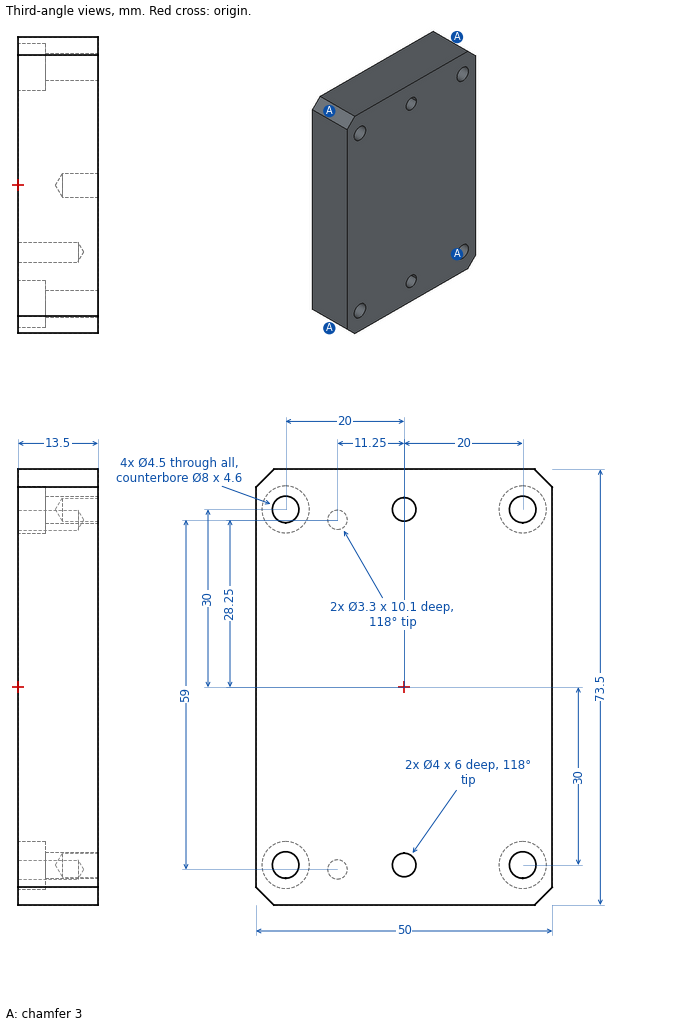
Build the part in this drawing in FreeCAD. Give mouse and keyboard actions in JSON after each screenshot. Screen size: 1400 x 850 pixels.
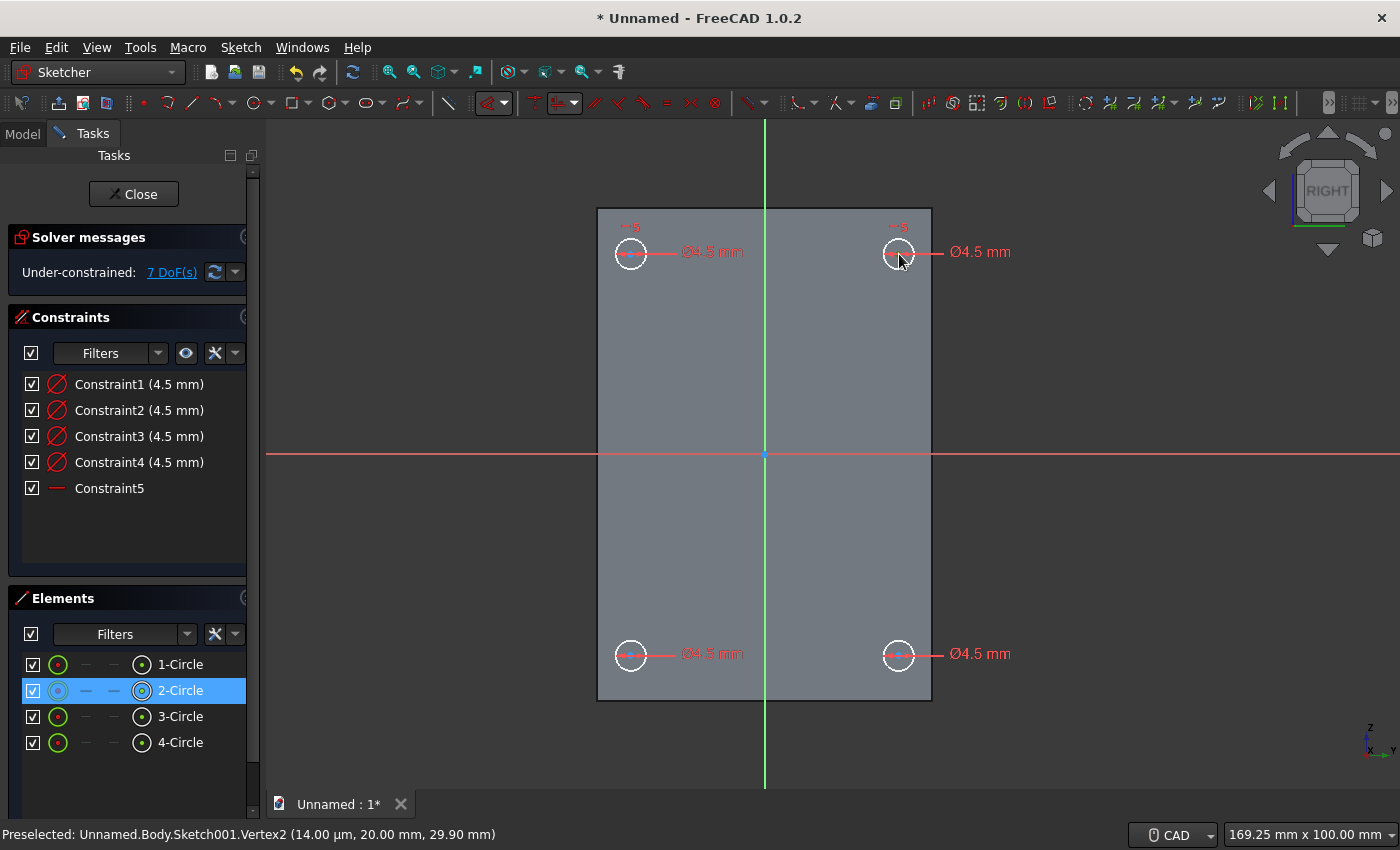
{"action": "left_click", "coordinate": [899, 656]}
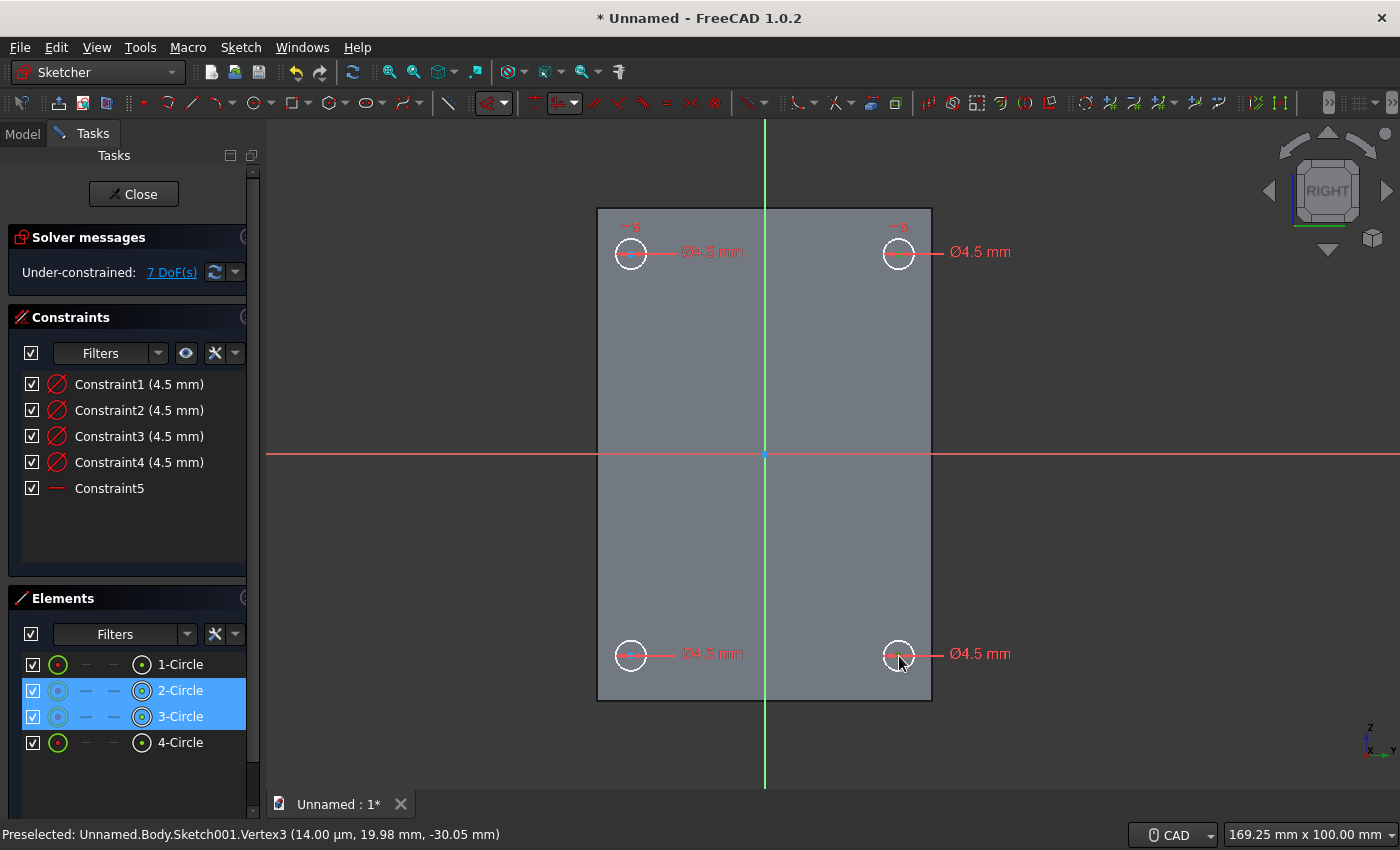
{"action": "key", "text": "v"}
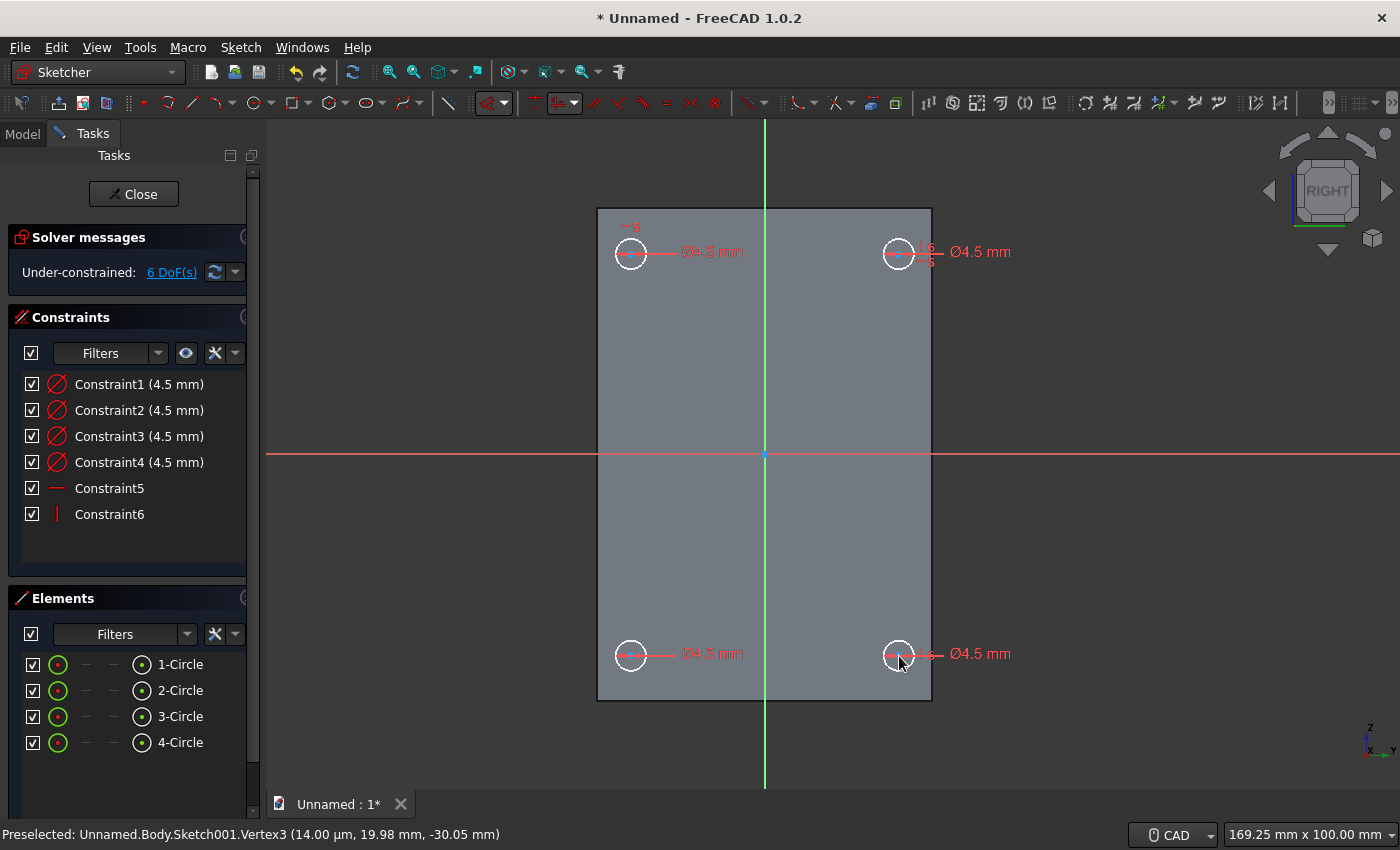
{"action": "left_click", "coordinate": [631, 254]}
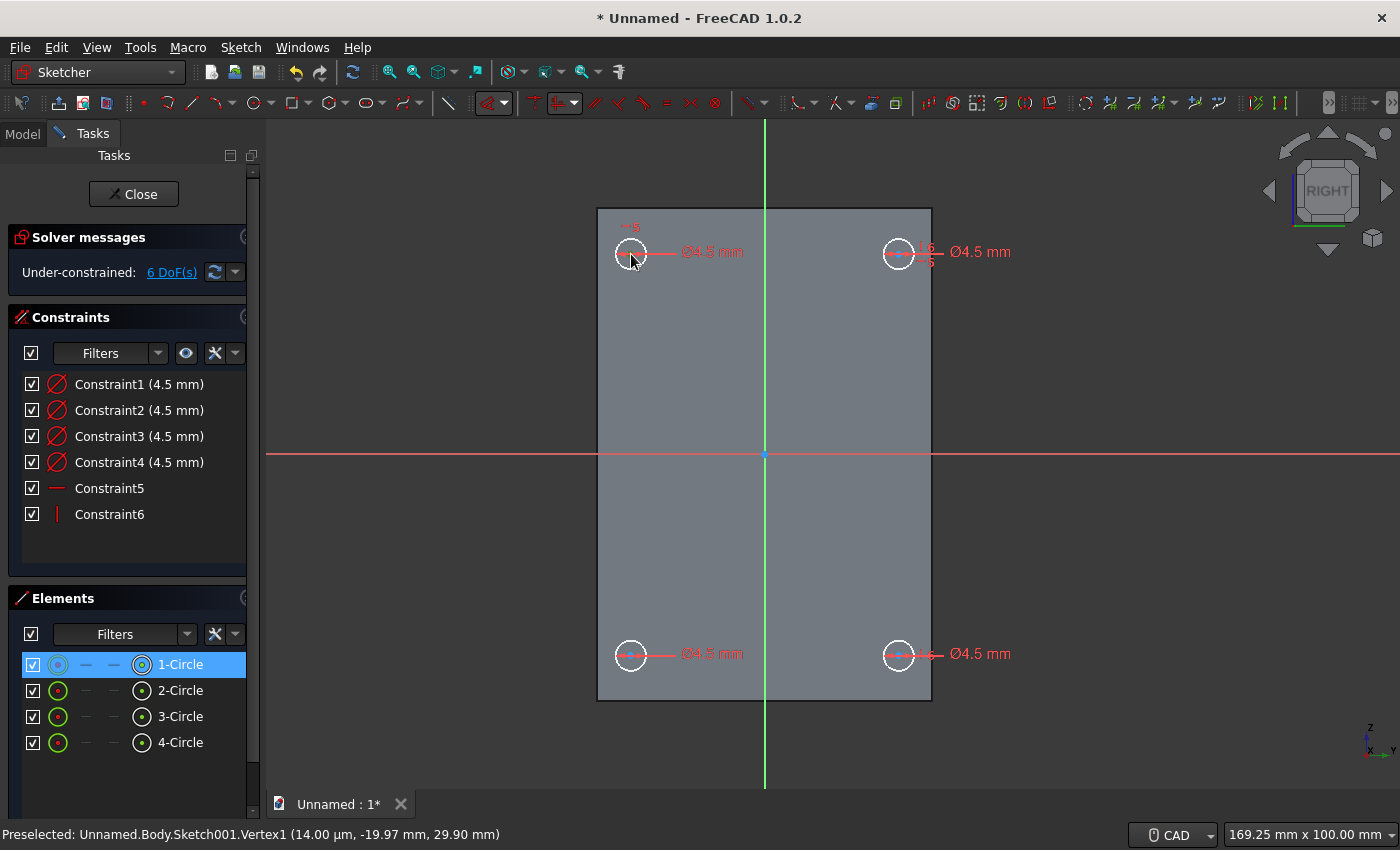
{"action": "left_click", "coordinate": [631, 656]}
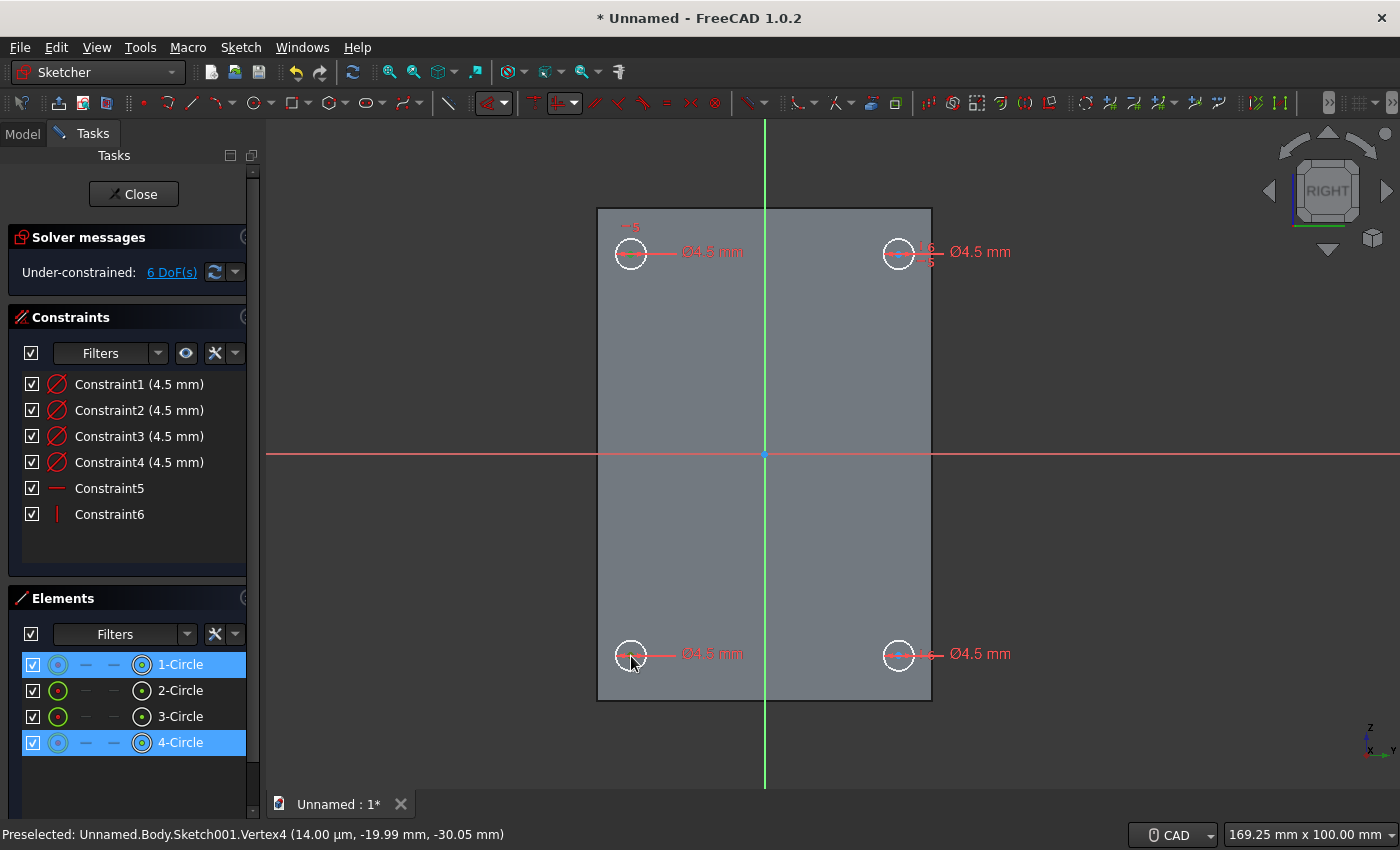
{"action": "left_click", "coordinate": [576, 104]}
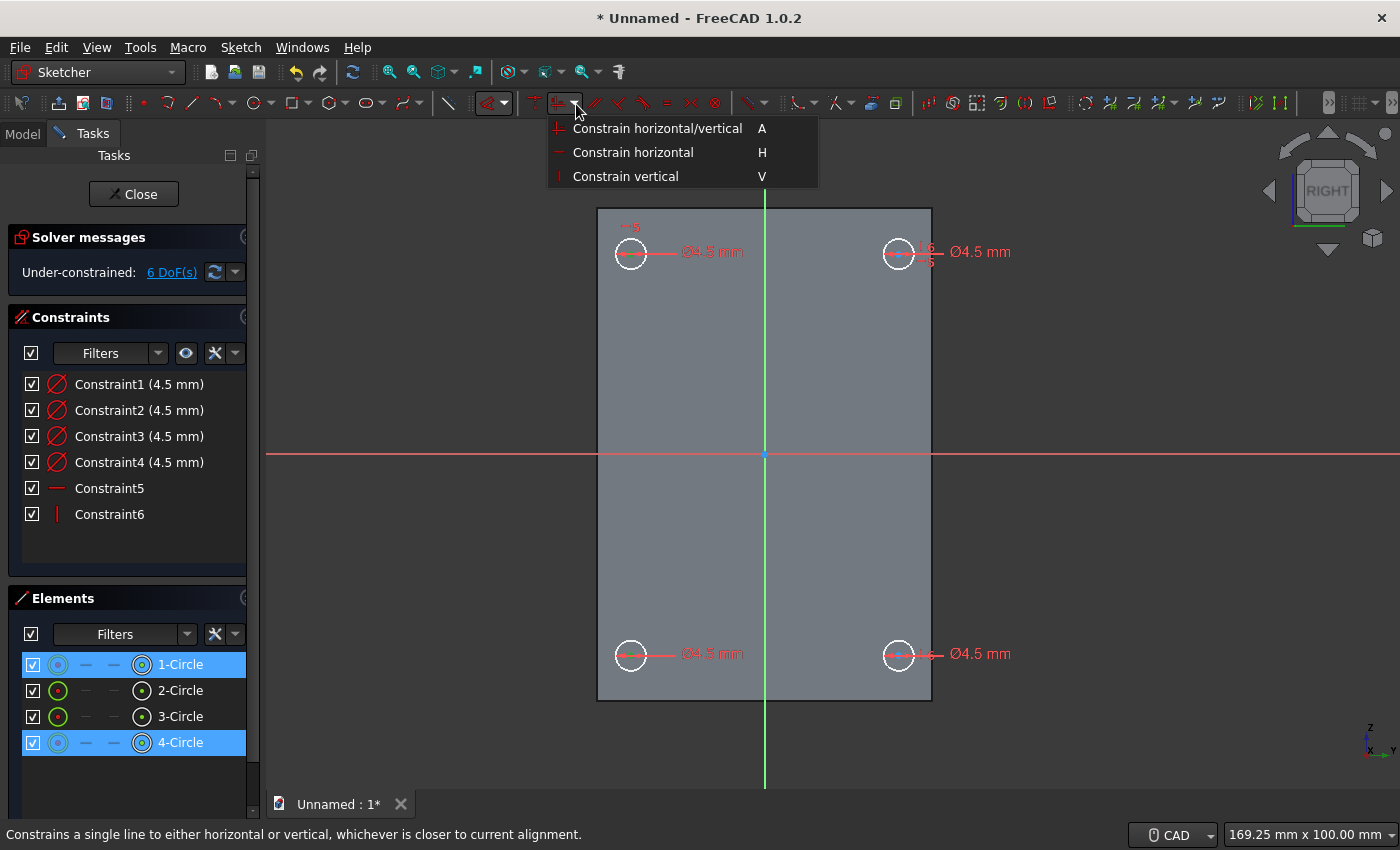
{"action": "left_click", "coordinate": [683, 176]}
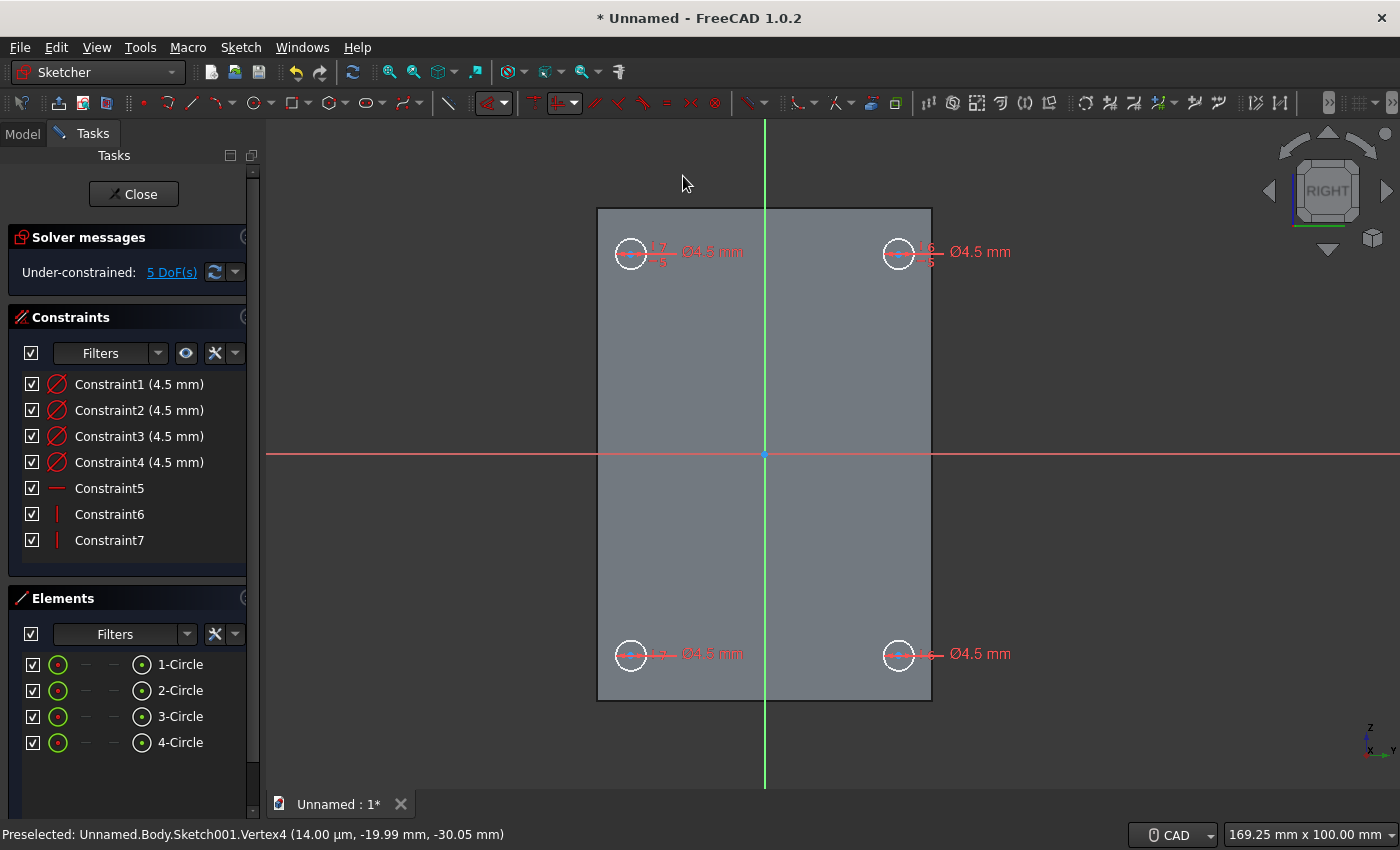
{"action": "left_click", "coordinate": [899, 656]}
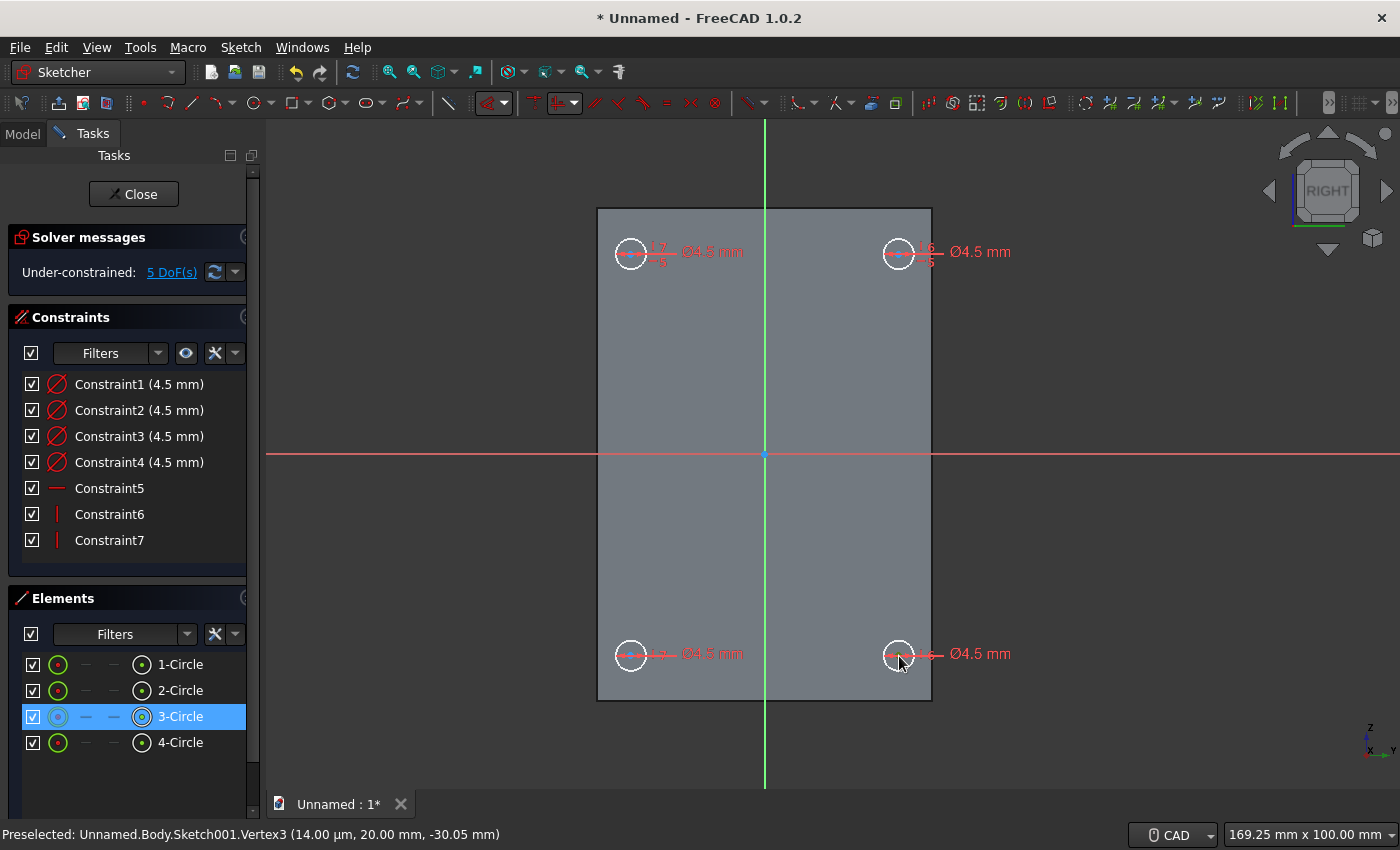
{"action": "left_click", "coordinate": [631, 656]}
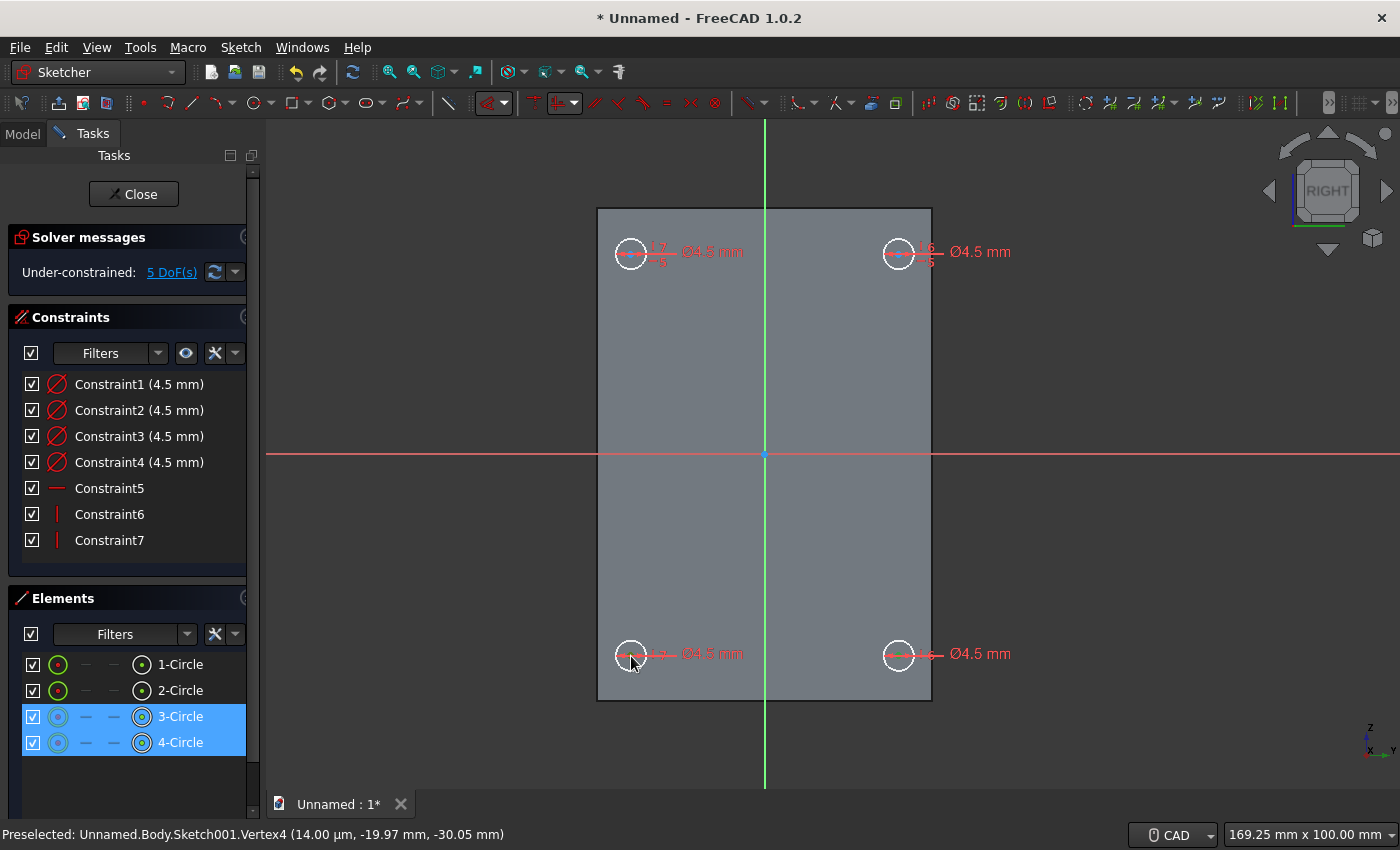
{"action": "left_click", "coordinate": [576, 104]}